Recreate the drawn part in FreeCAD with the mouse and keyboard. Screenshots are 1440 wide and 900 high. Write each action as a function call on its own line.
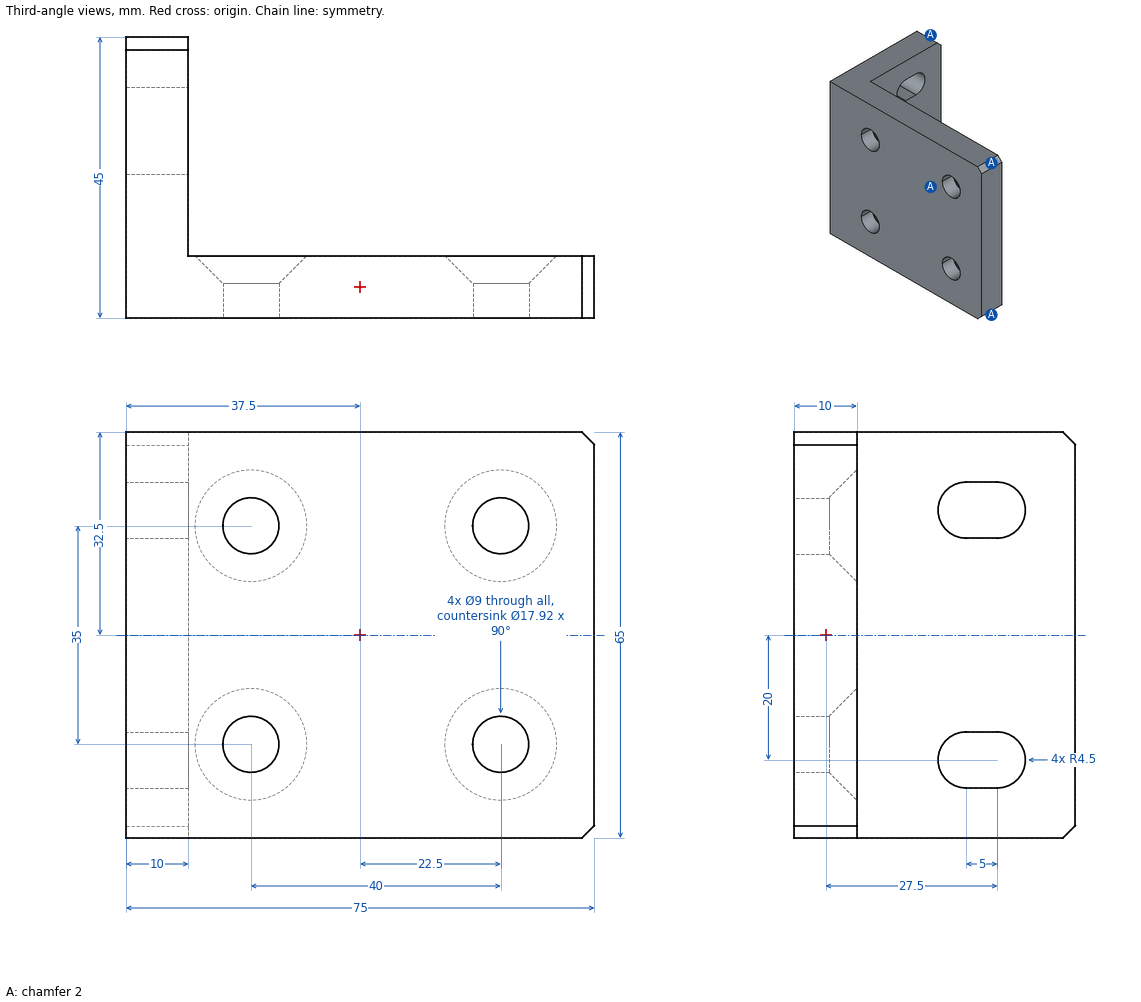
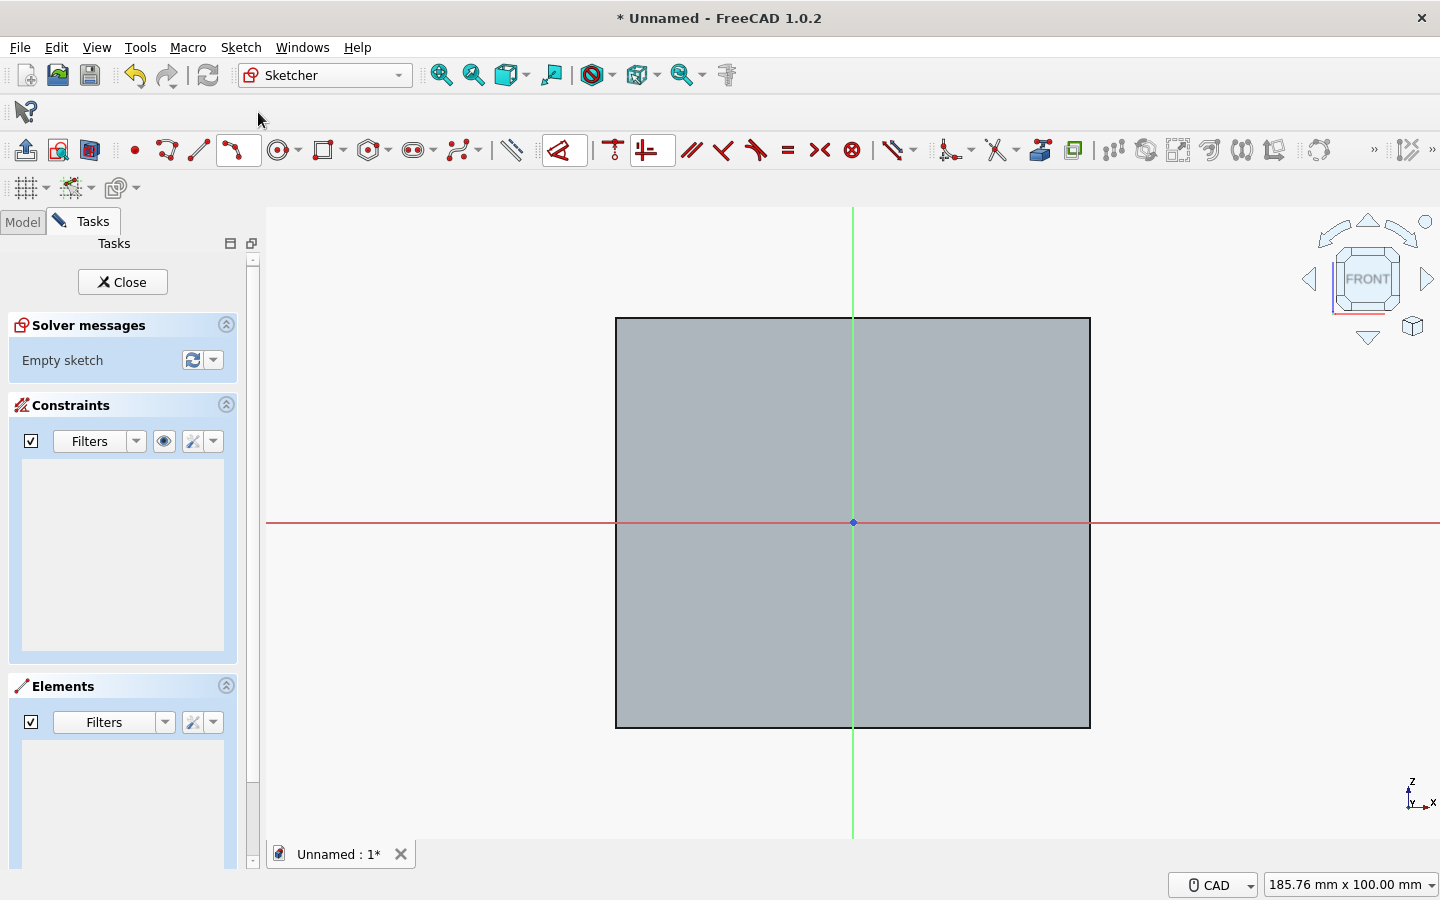
click(324, 150)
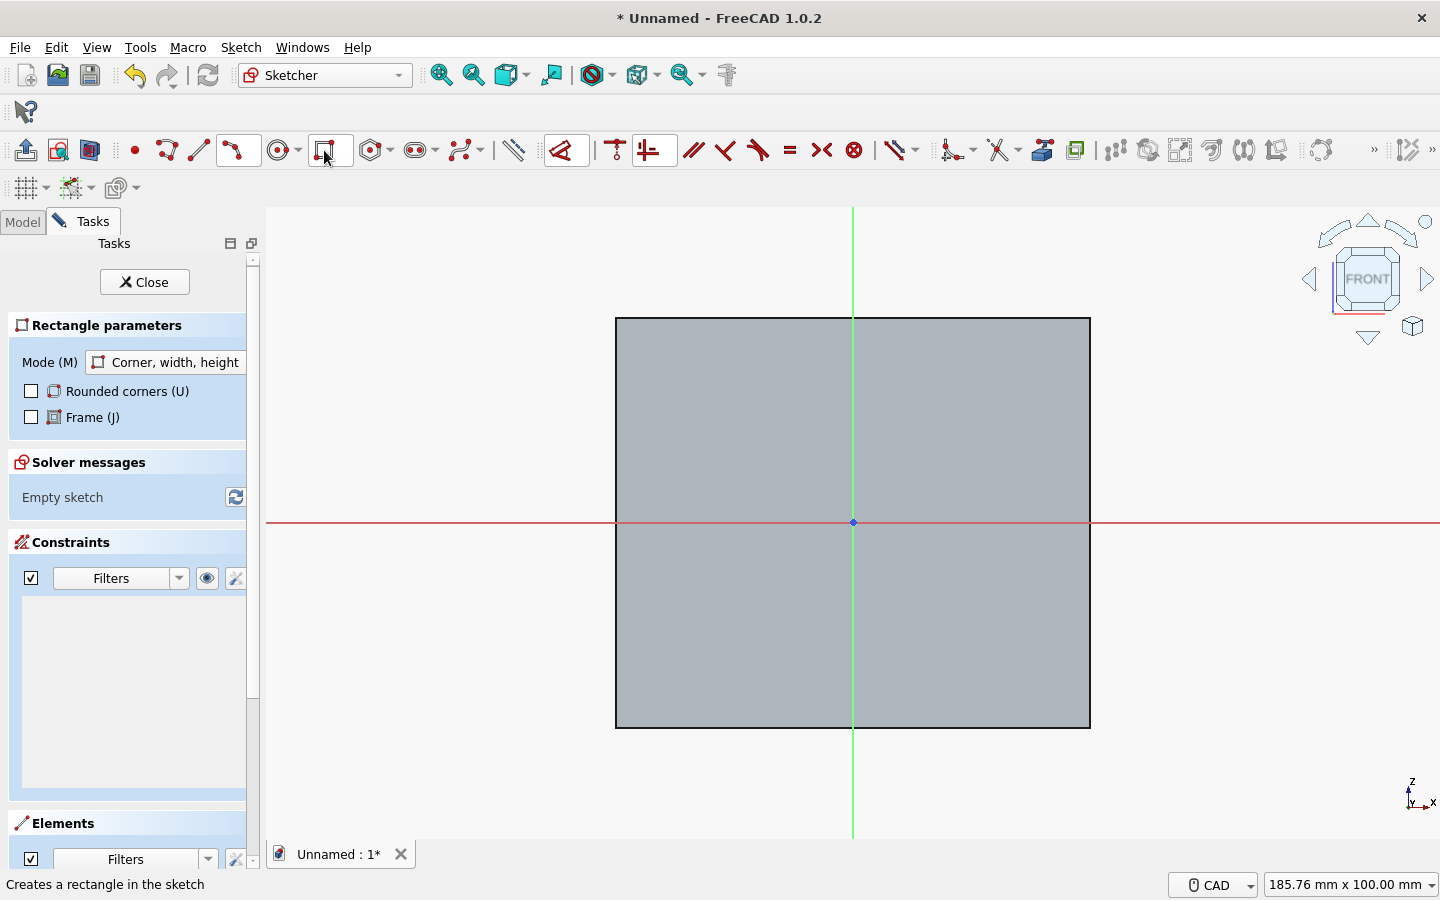
click(616, 318)
move(679, 728)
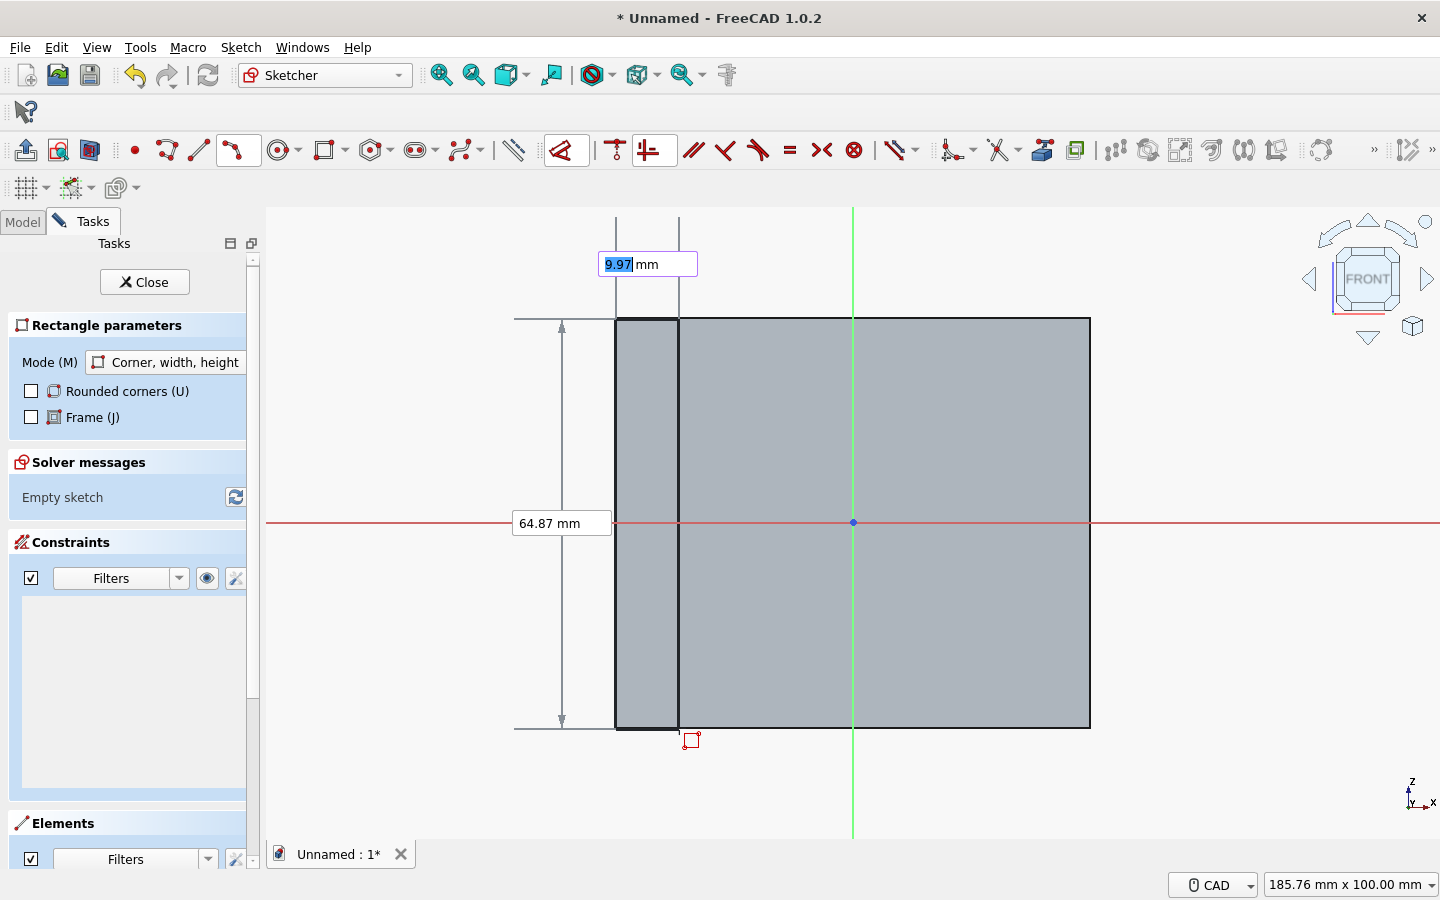
text(10)
key(Tab)
text(65)
key(Return)
key(Escape)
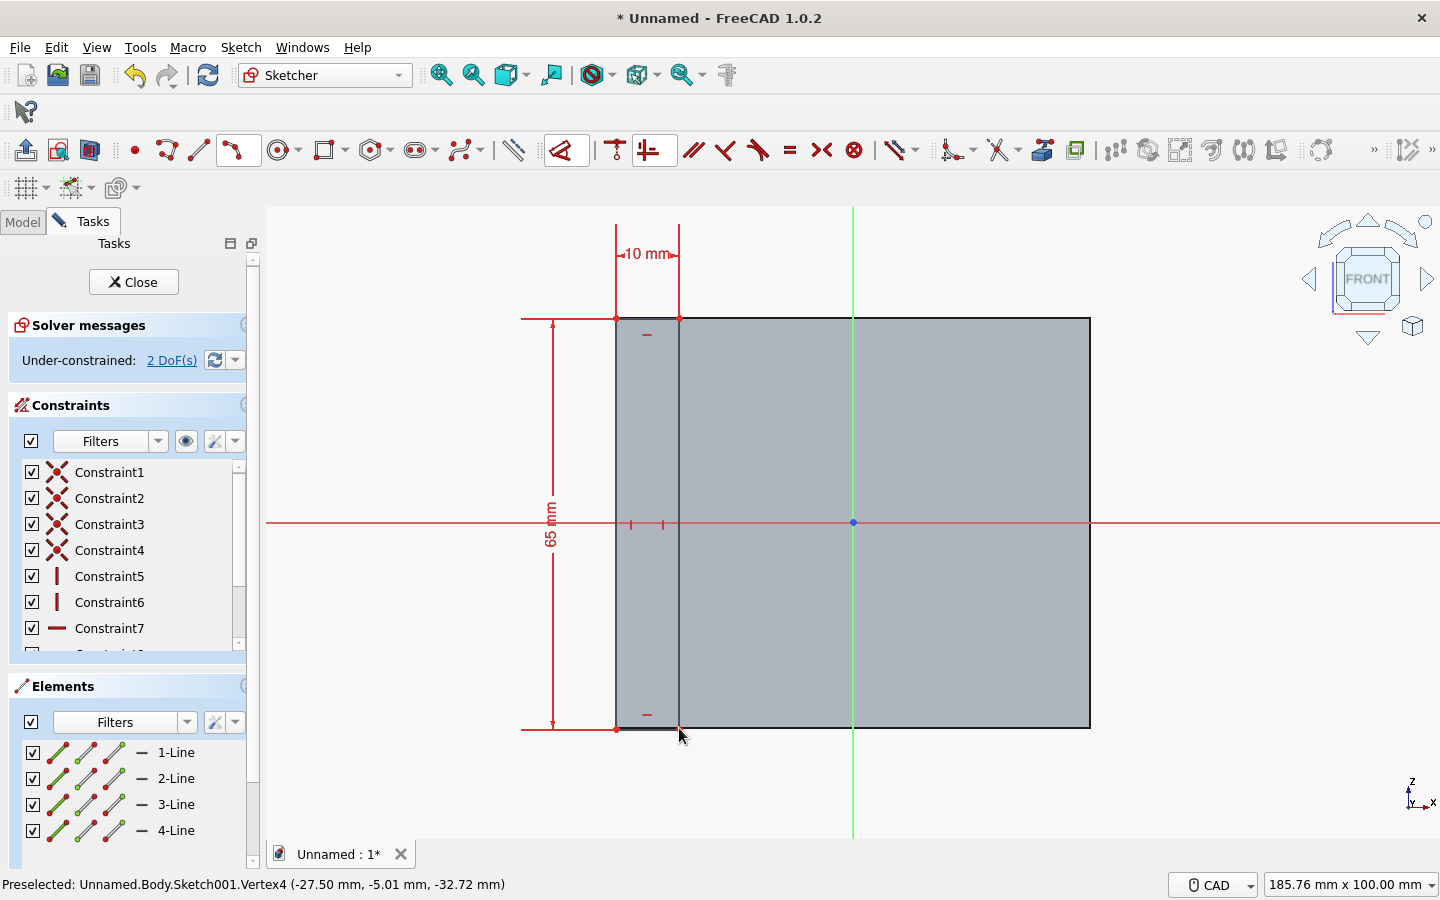
key(d)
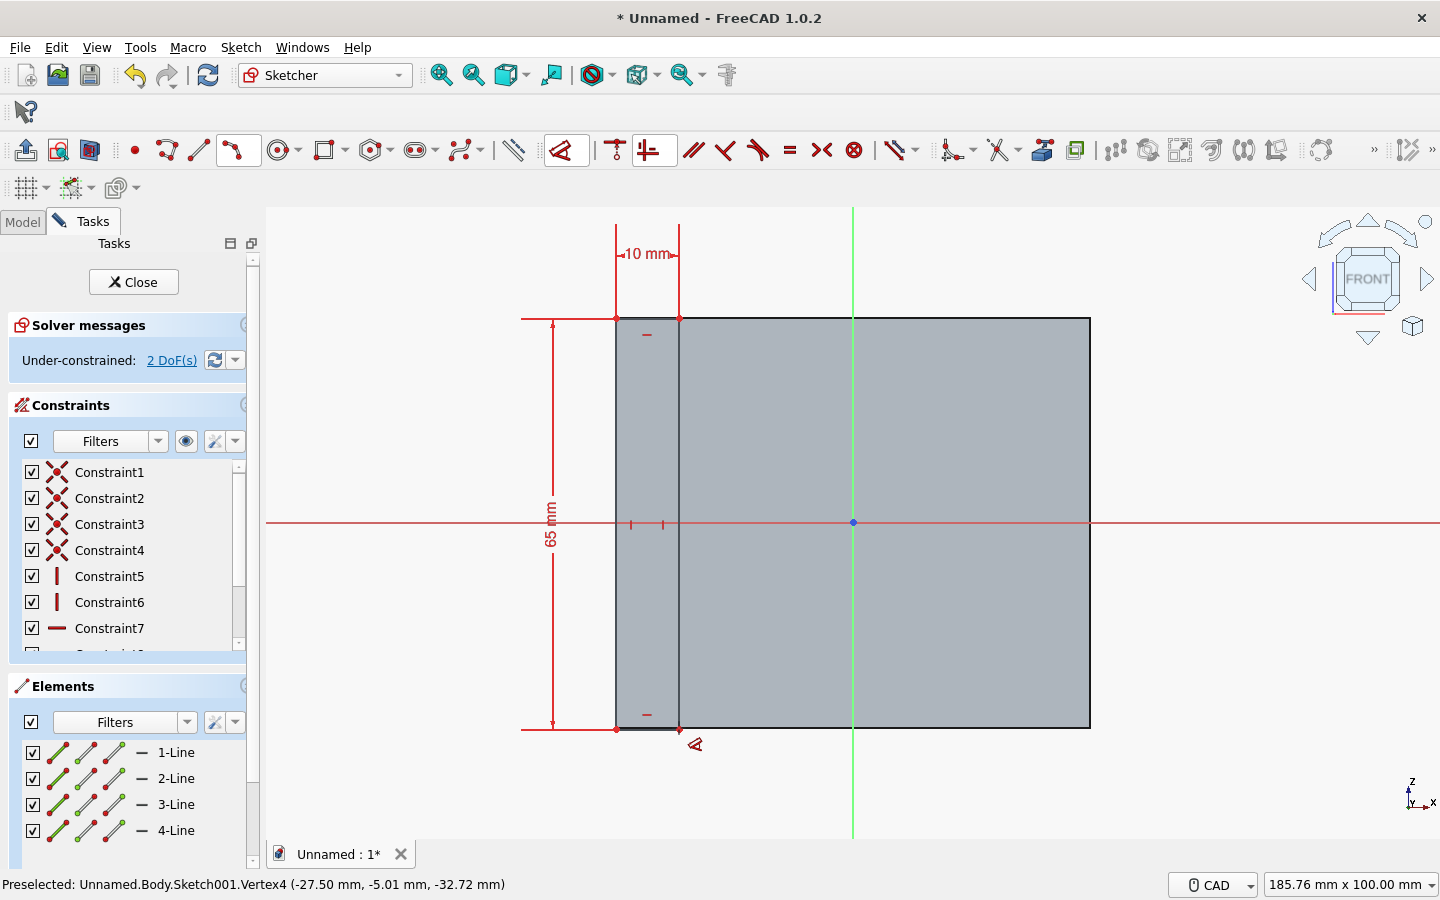
click(616, 319)
click(734, 285)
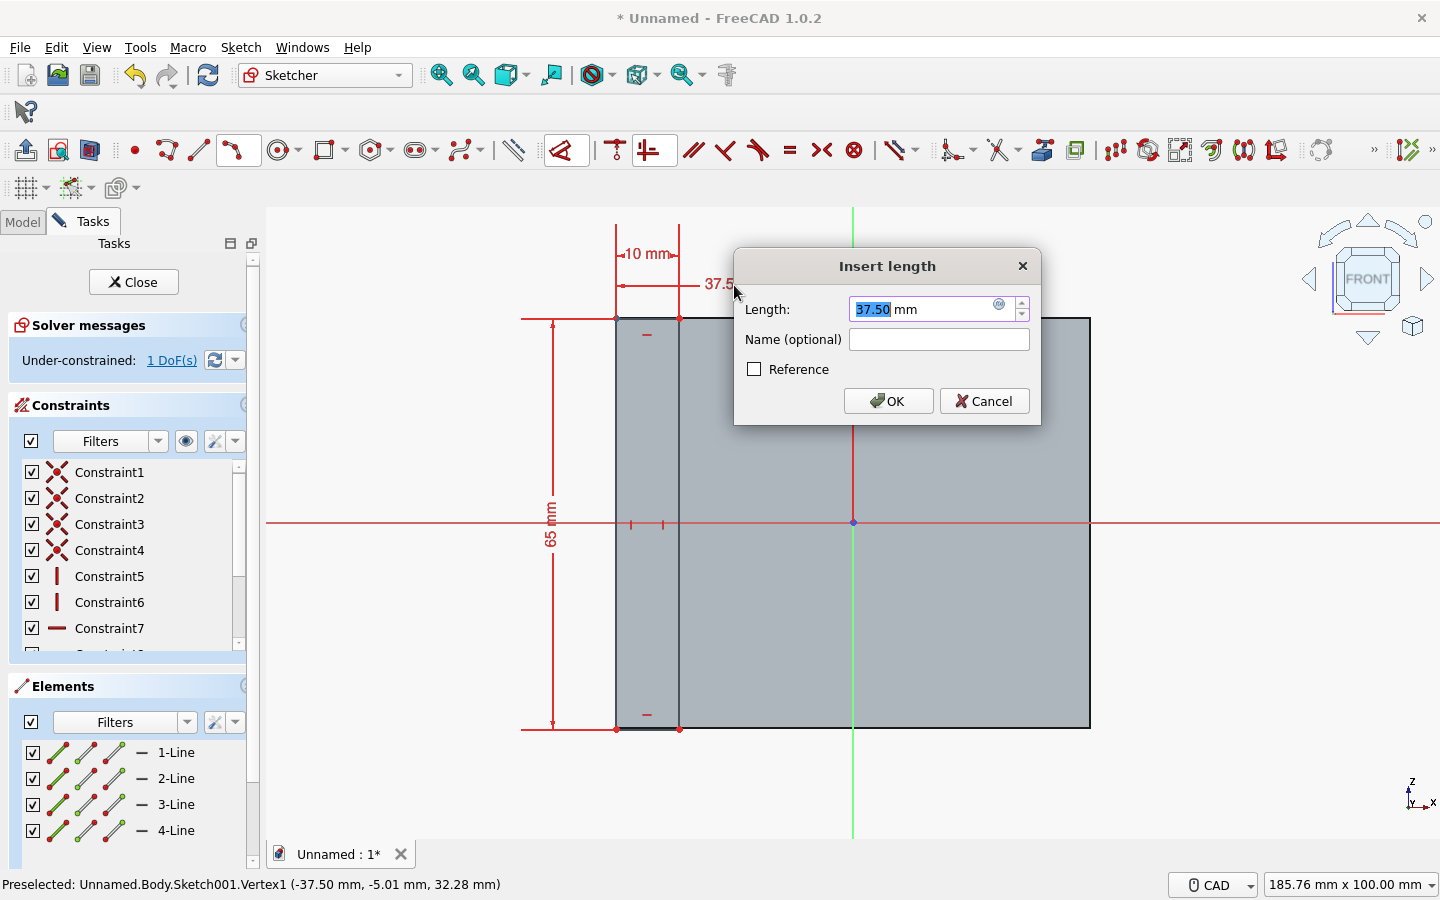
text(37.5)
key(Return)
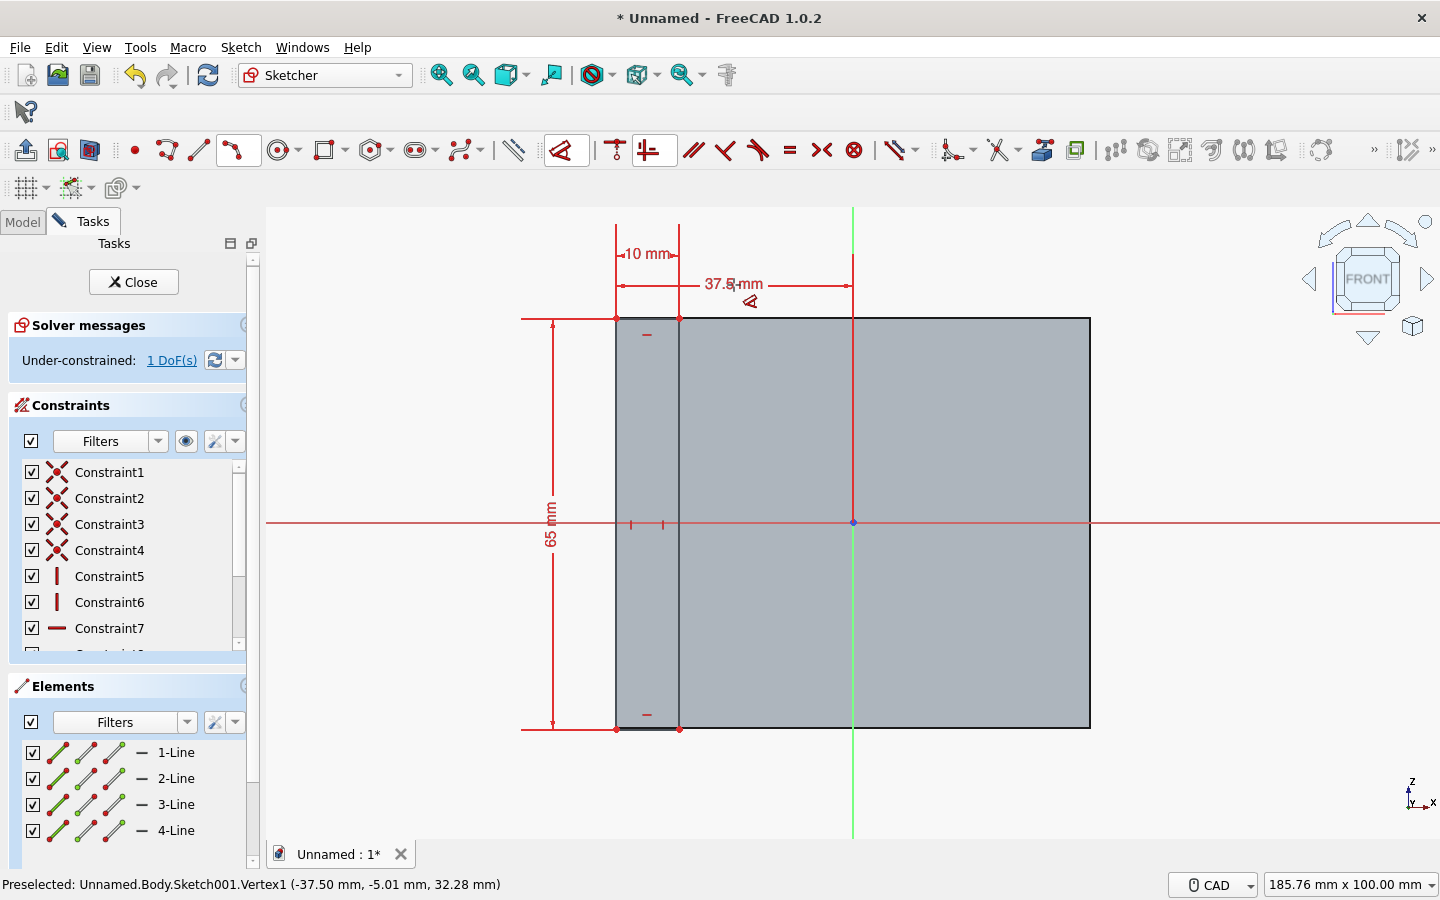
click(616, 319)
click(887, 421)